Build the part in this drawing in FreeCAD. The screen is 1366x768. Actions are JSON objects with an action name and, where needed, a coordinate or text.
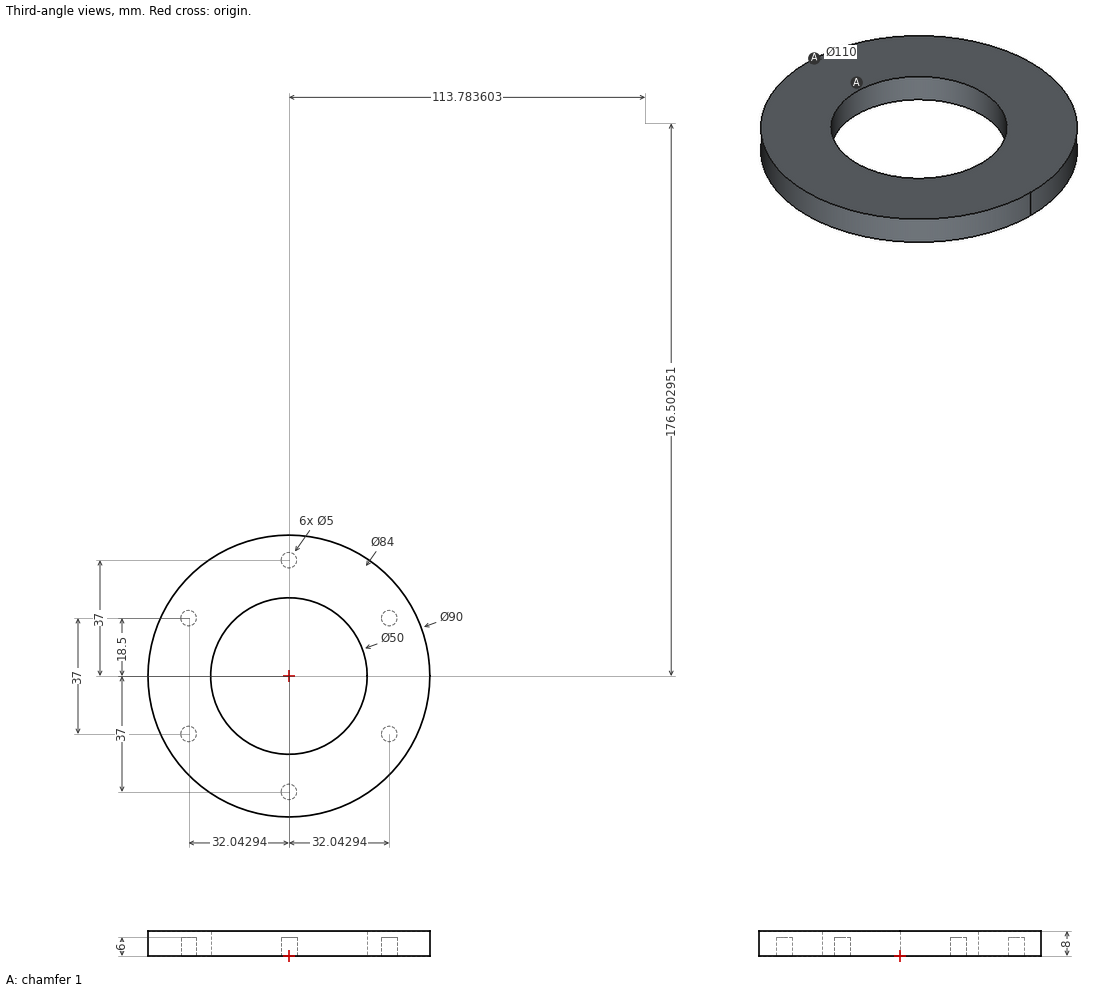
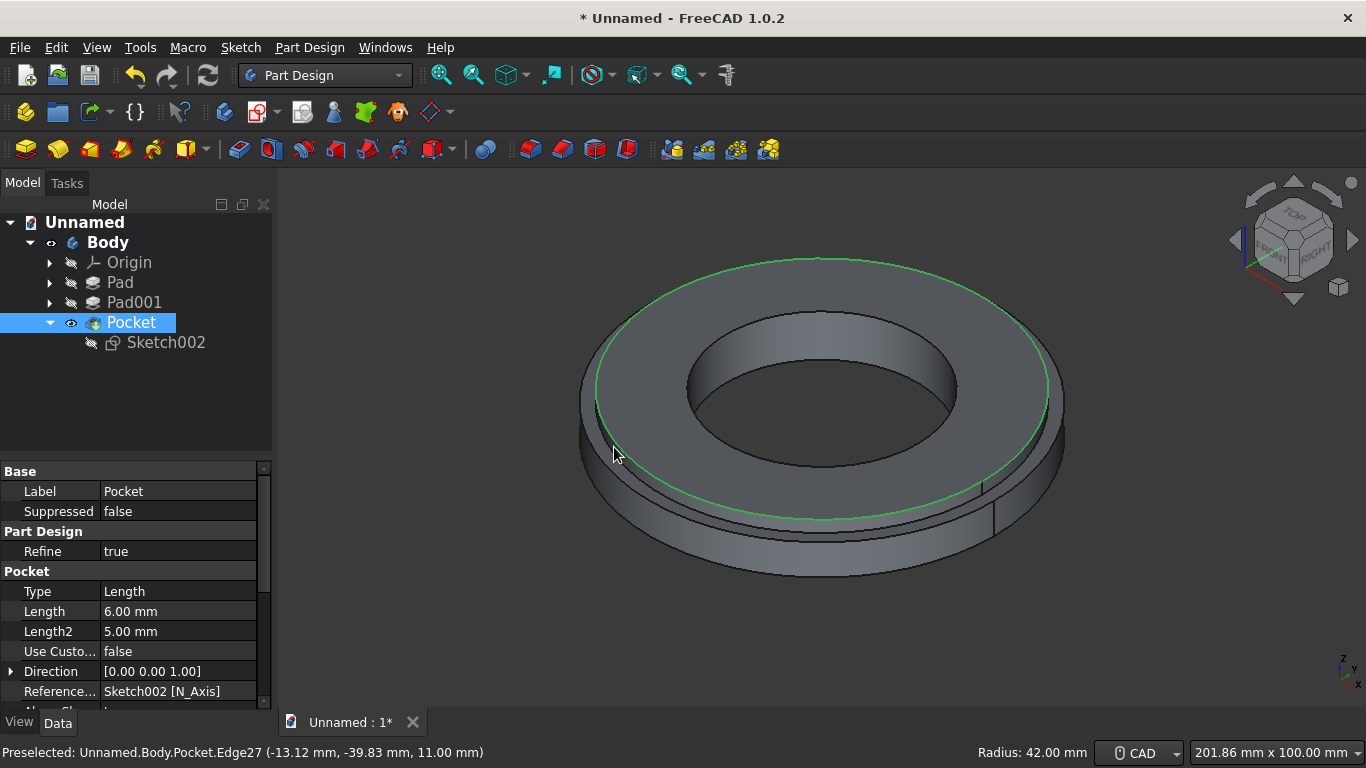
{"action": "left_click", "coordinate": [727, 333], "text": "ctrl"}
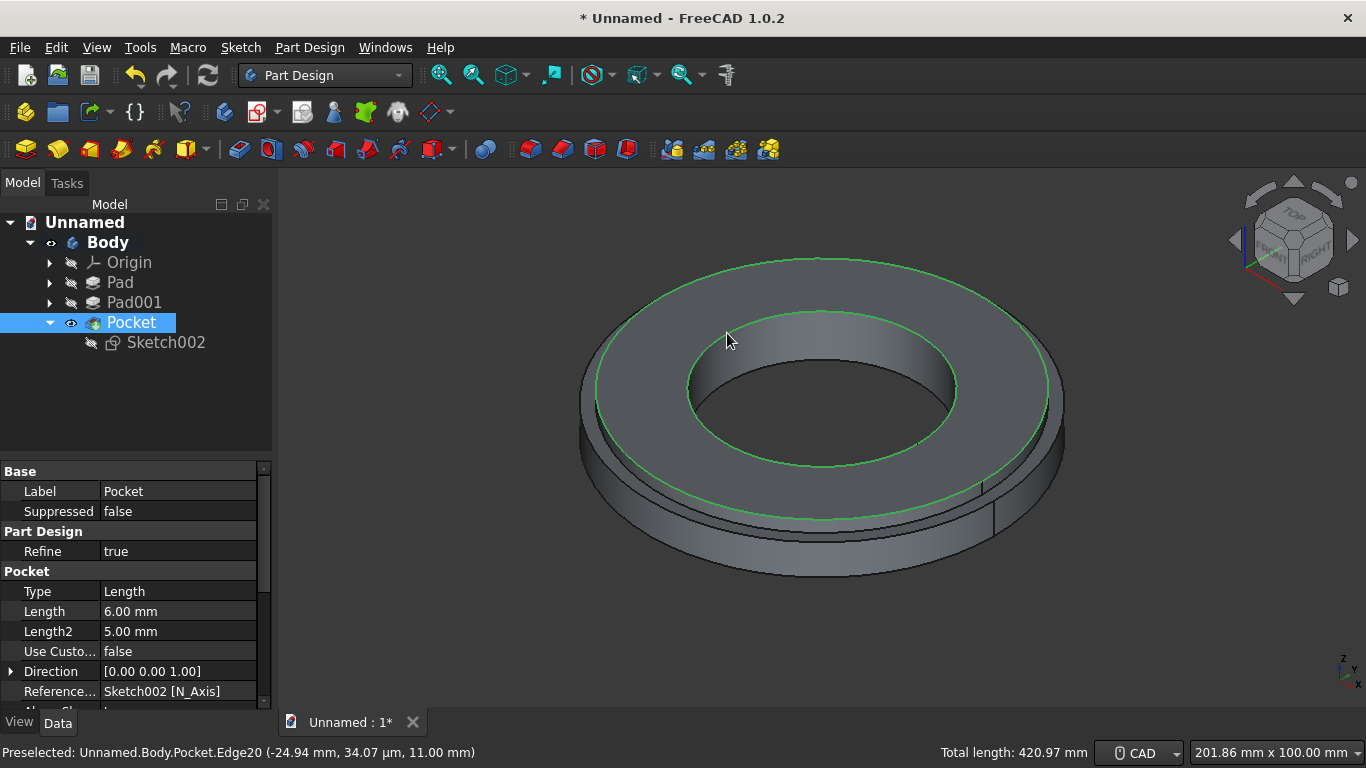
{"action": "left_click", "coordinate": [564, 150]}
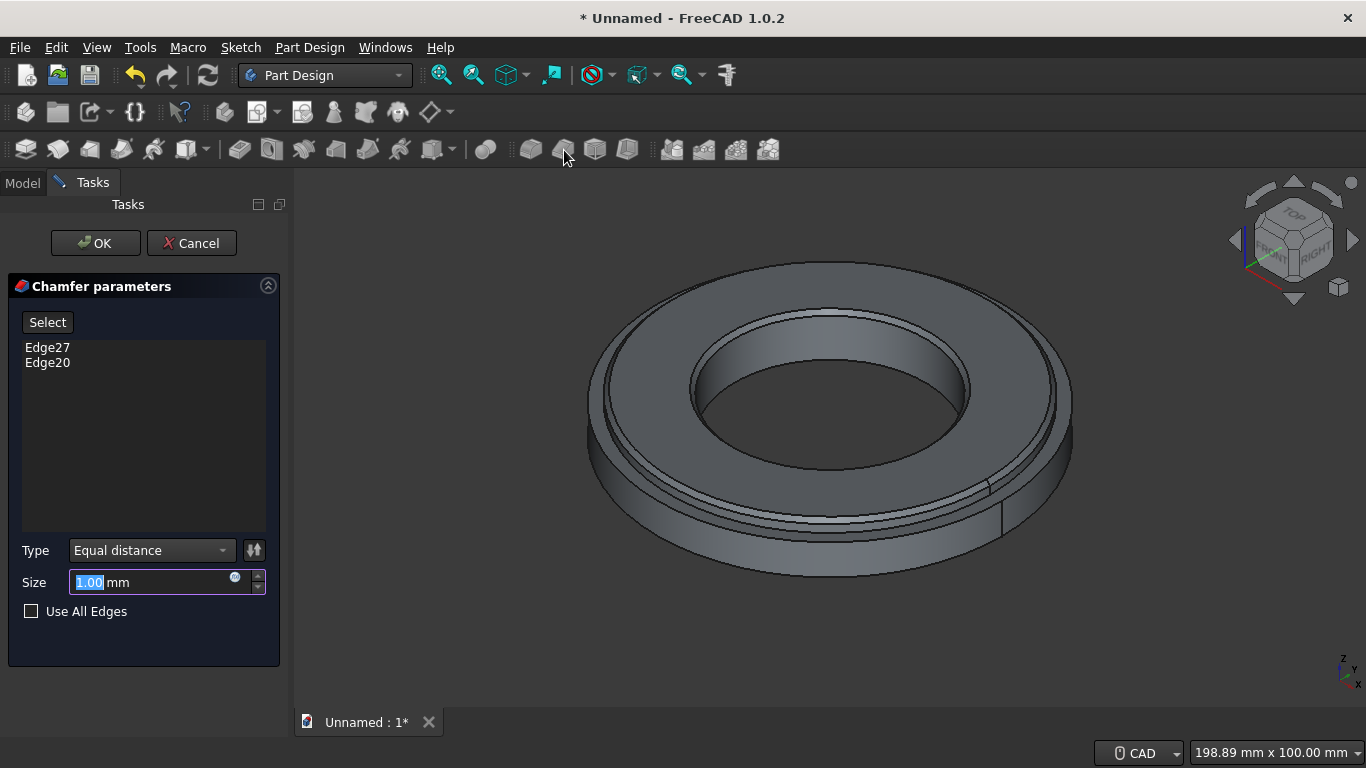
{"action": "type", "text": "1"}
{"action": "key", "text": "Tab"}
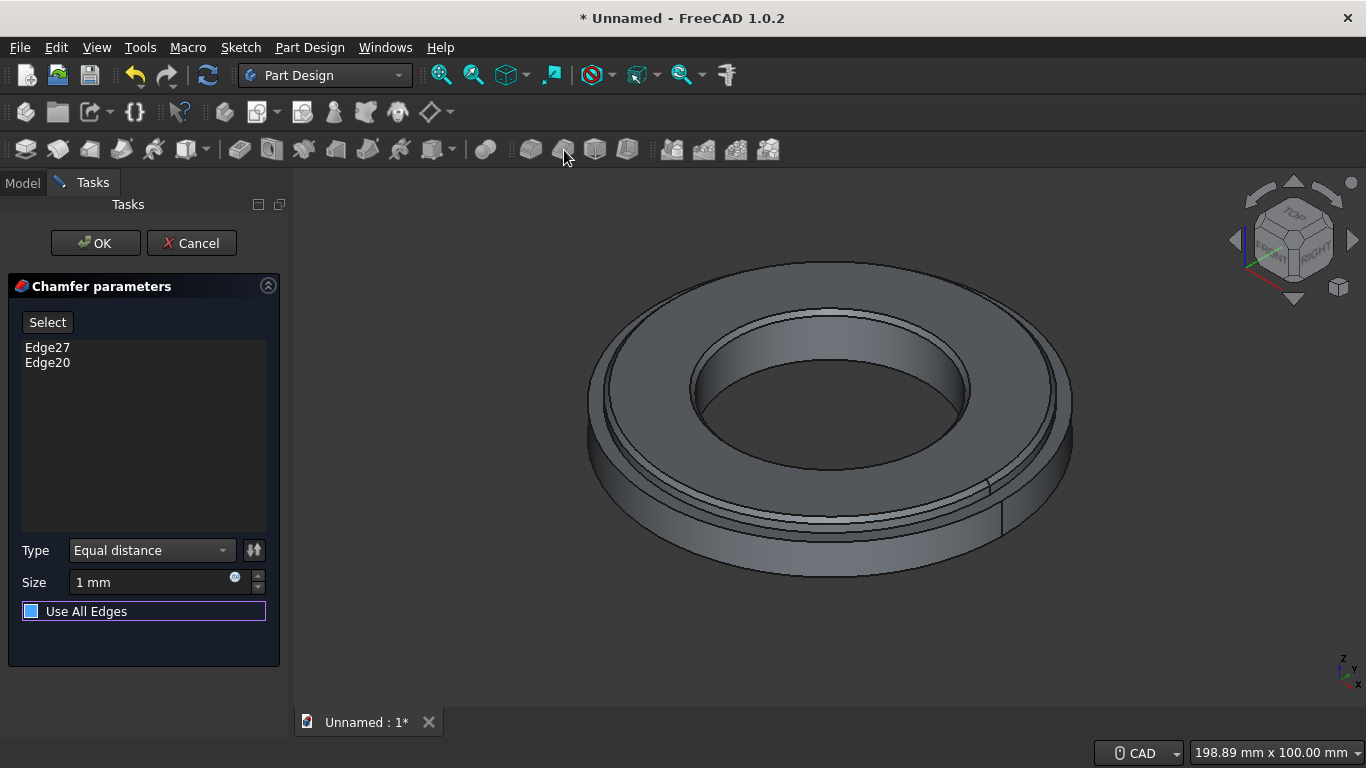
{"action": "left_click", "coordinate": [96, 243]}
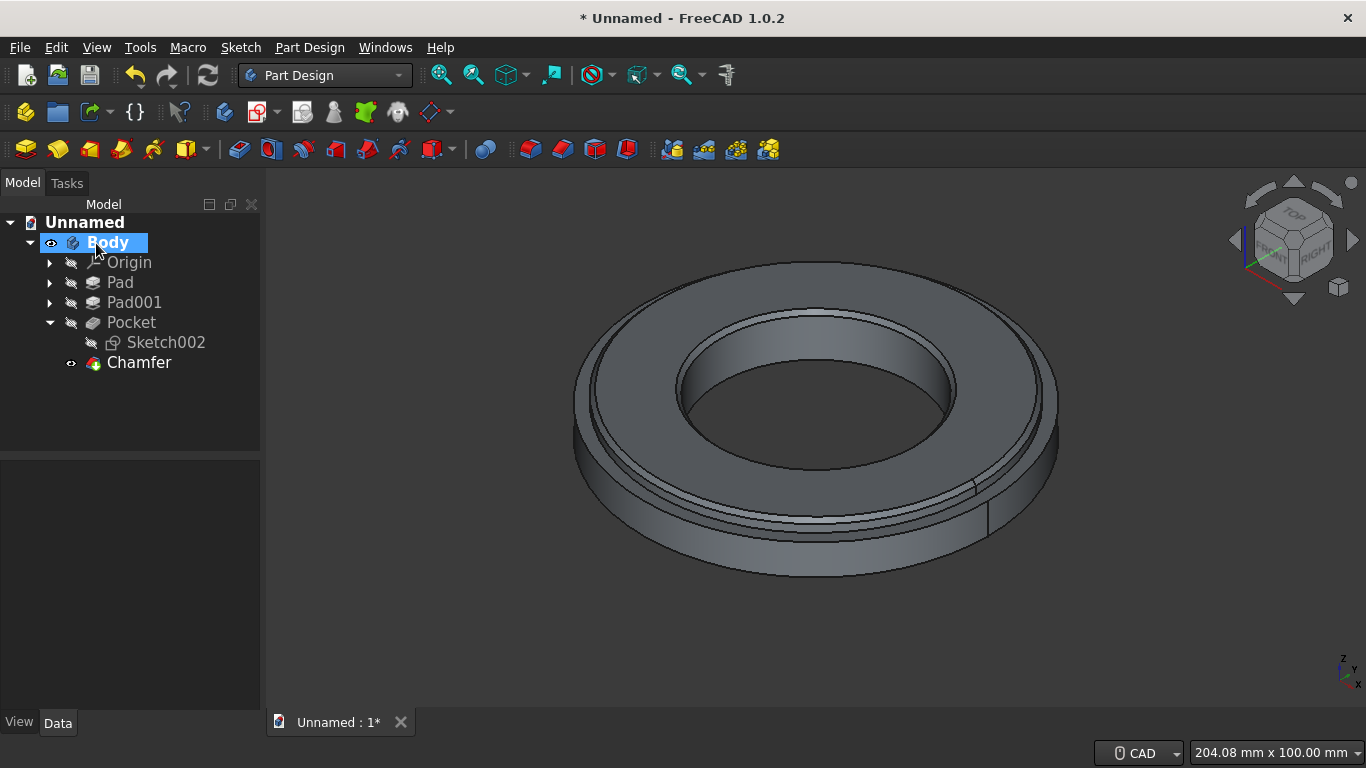
{"action": "left_click", "coordinate": [1052, 388]}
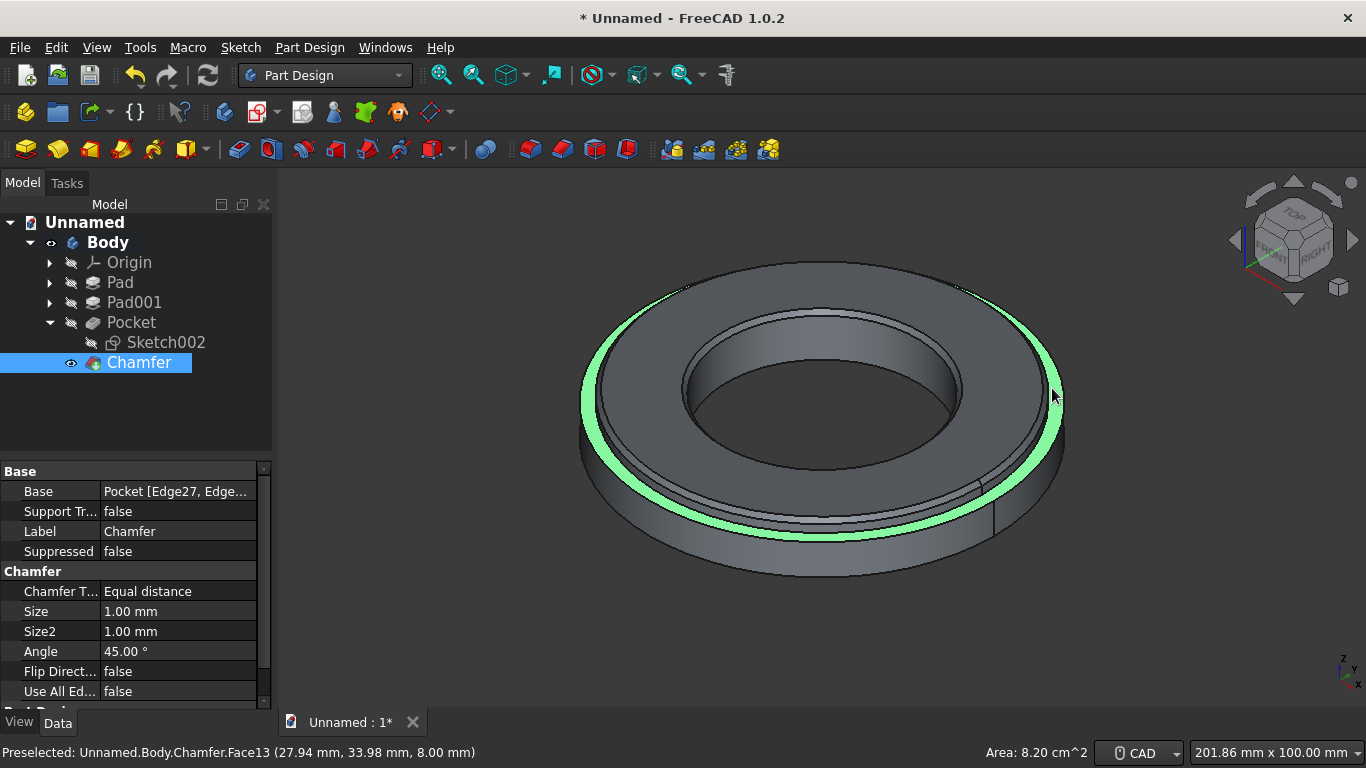
{"action": "left_click", "coordinate": [258, 112]}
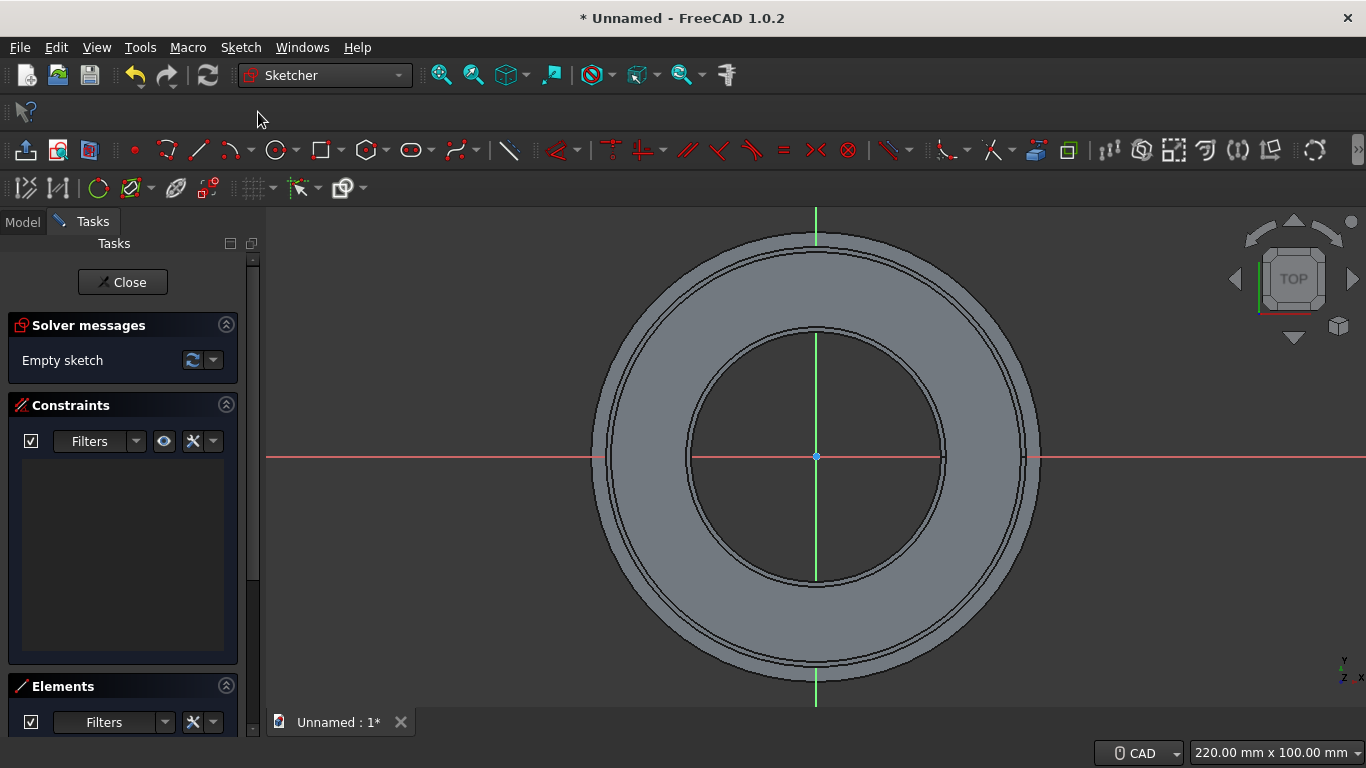
{"action": "scroll", "coordinate": [621, 612], "scroll_direction": "down", "scroll_amount": 7}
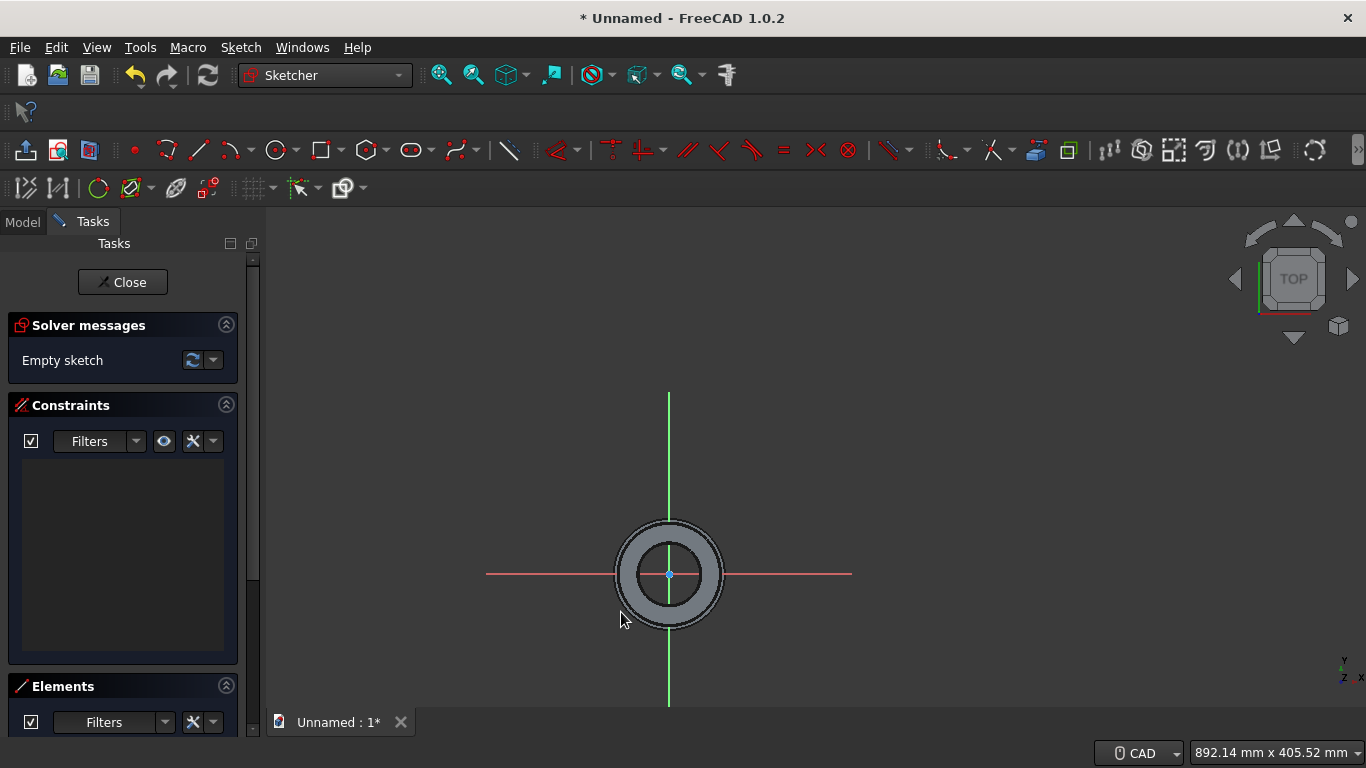
{"action": "key", "text": "g c"}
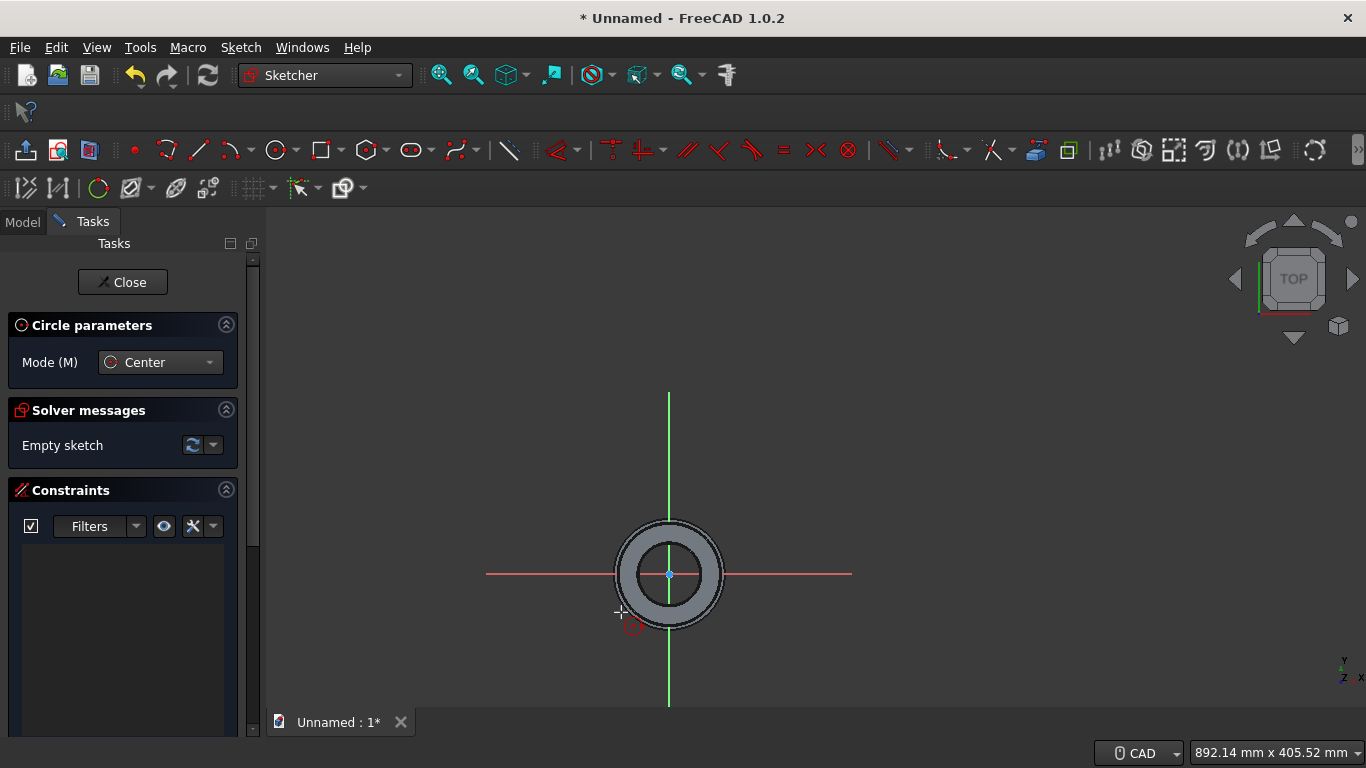
{"action": "left_click", "coordinate": [669, 574]}
{"action": "mouse_move", "coordinate": [706, 538]}